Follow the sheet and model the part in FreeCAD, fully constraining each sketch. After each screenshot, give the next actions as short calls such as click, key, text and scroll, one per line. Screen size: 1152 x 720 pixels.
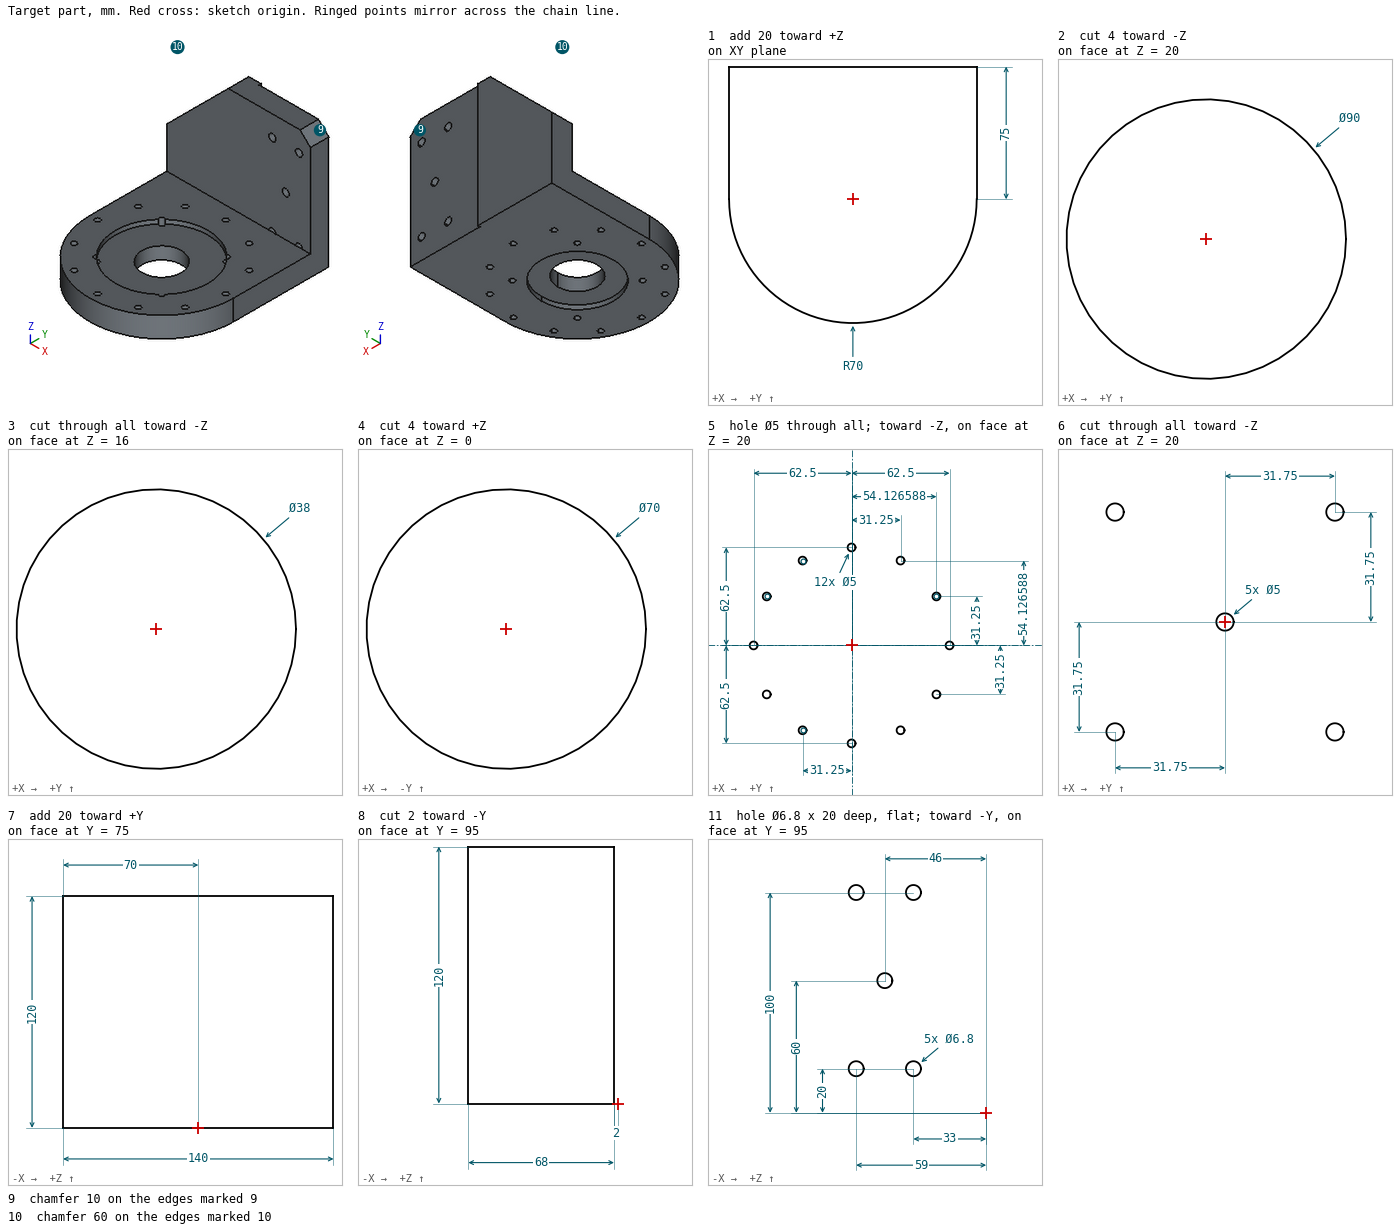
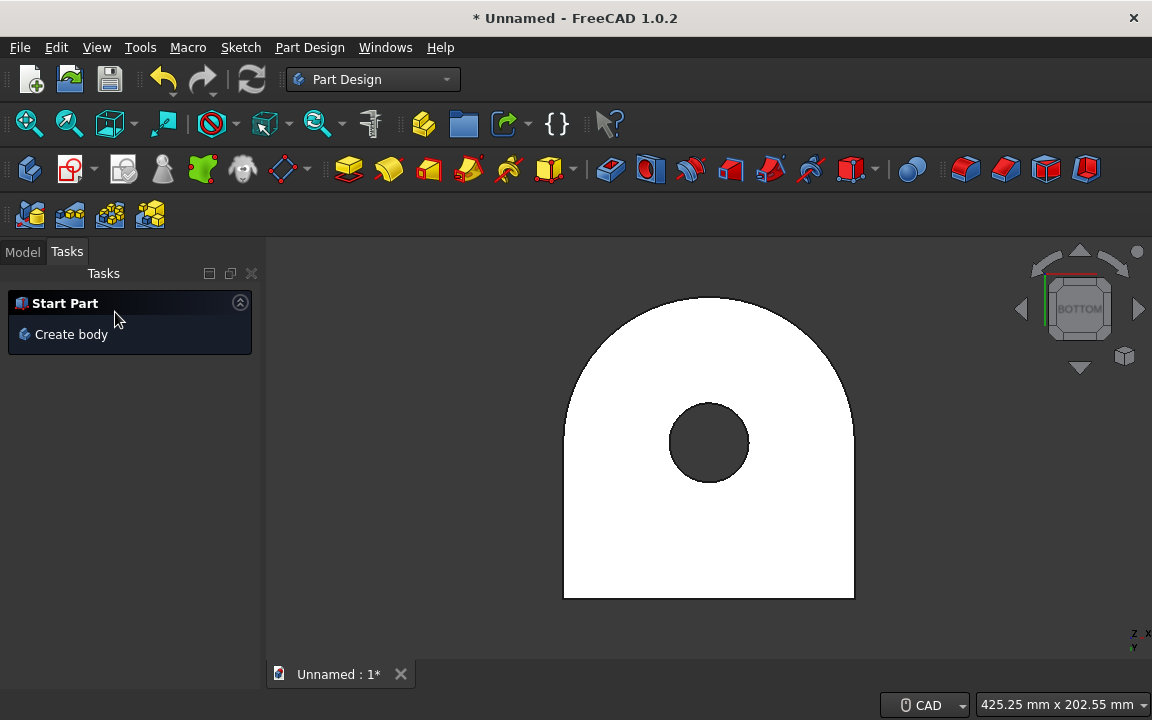
click(792, 533)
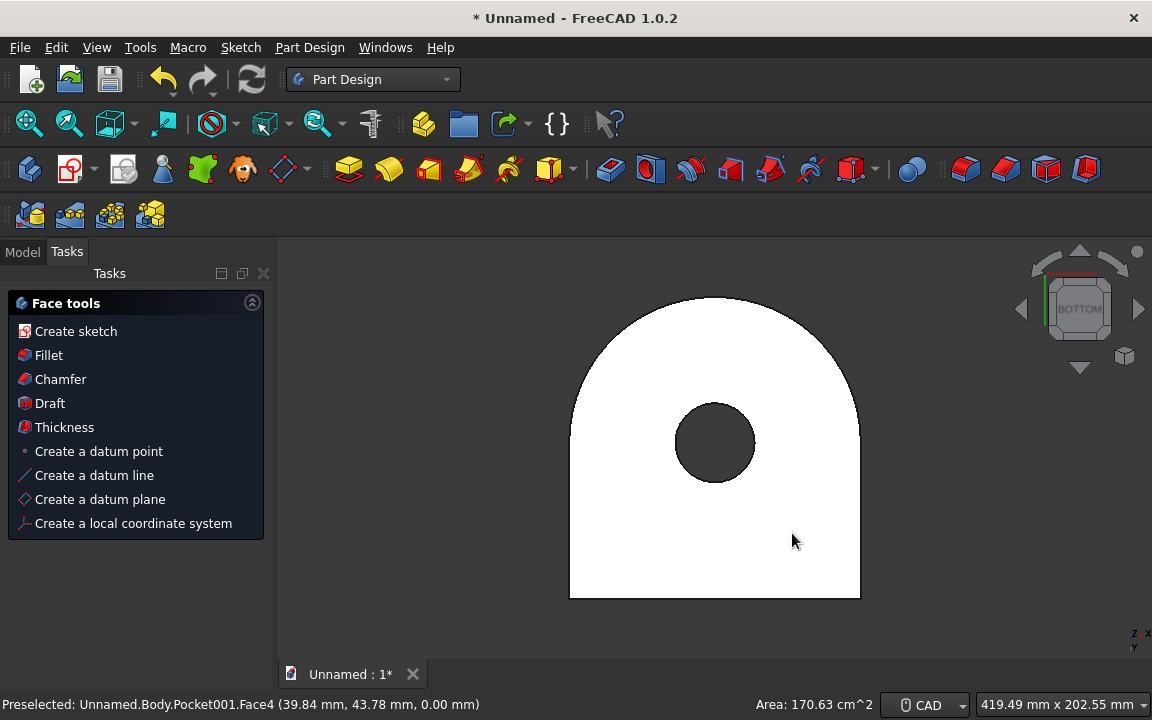
click(70, 170)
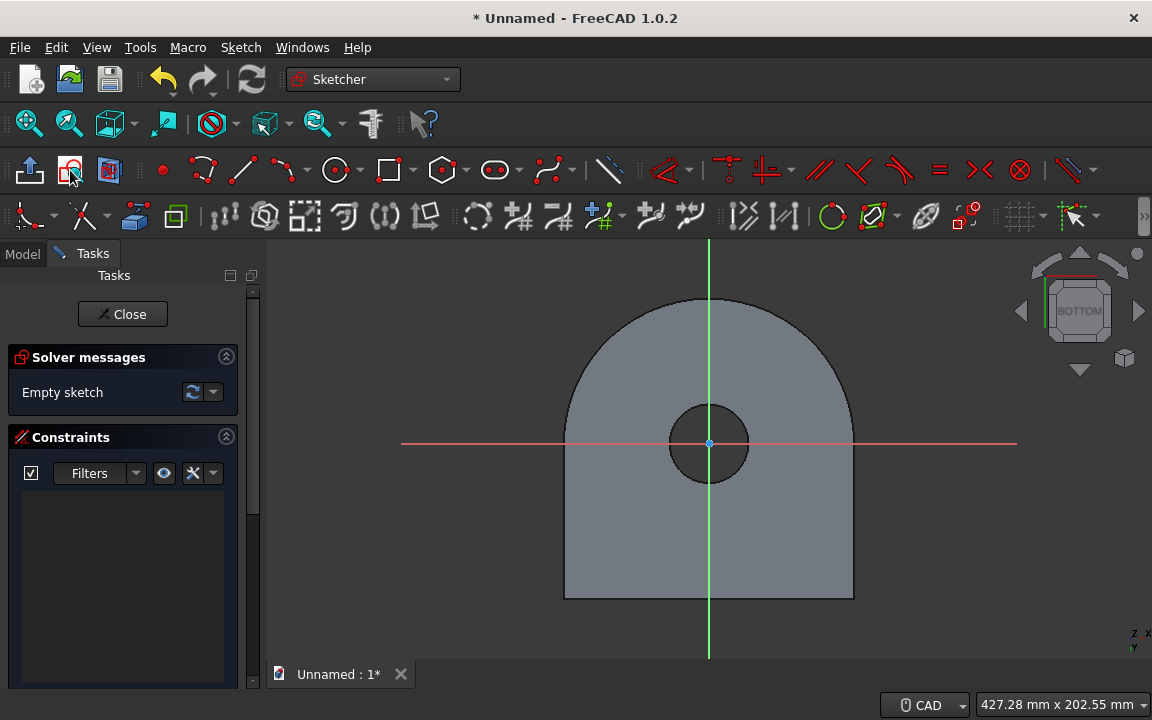
scroll(792, 438, up, 3)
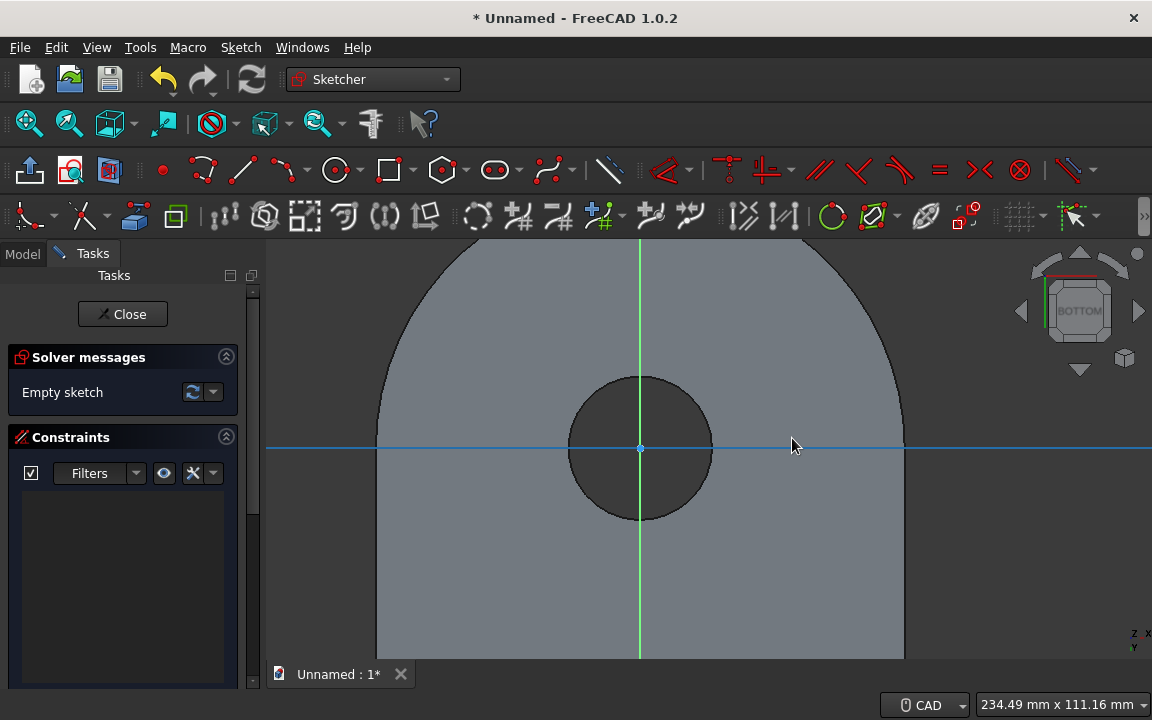
key(g)
key(c)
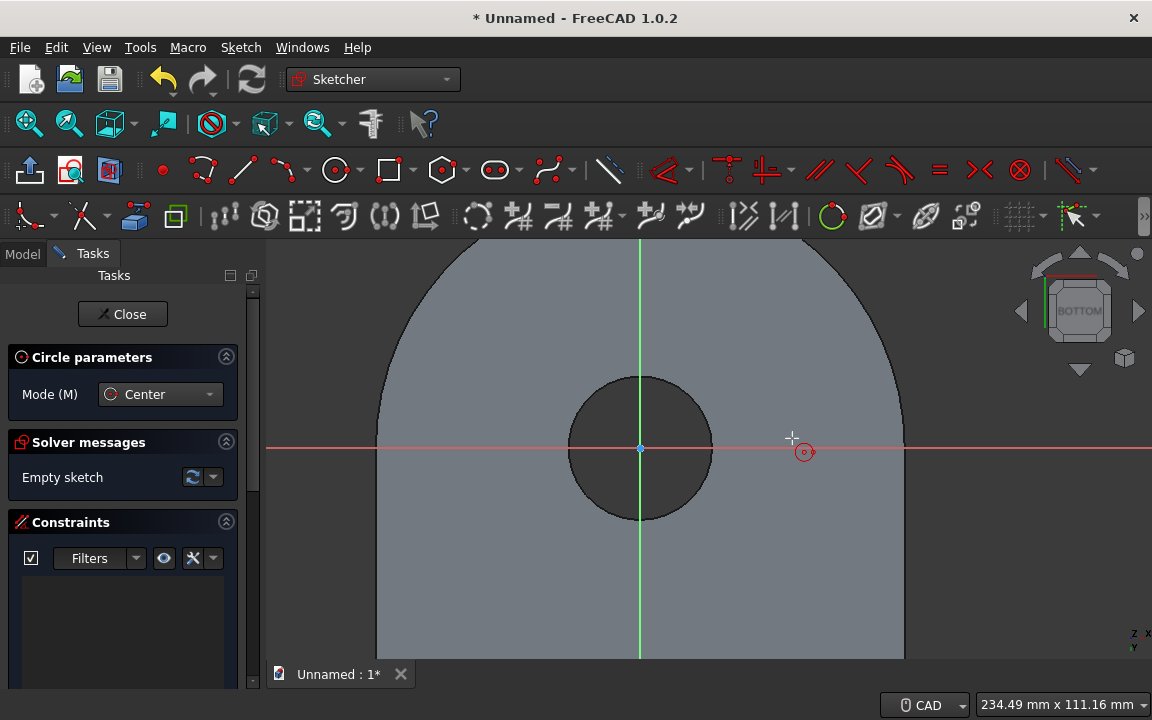
click(640, 448)
move(734, 355)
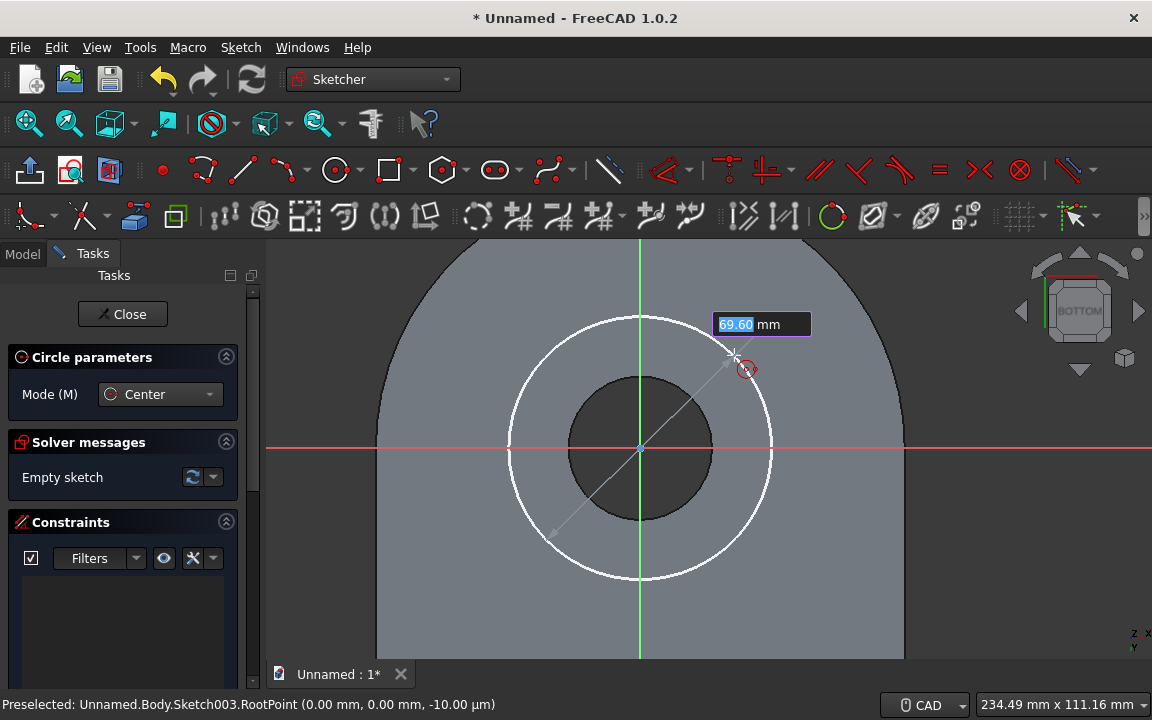
text(70)
key(Return)
key(Escape)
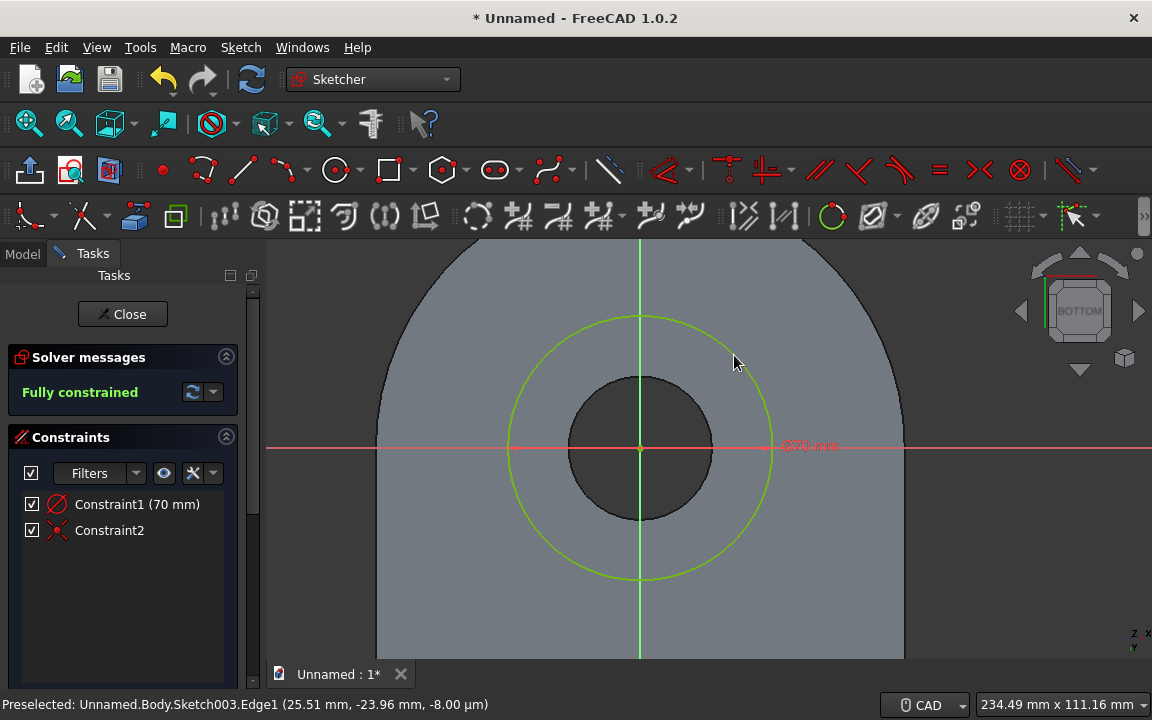
click(123, 314)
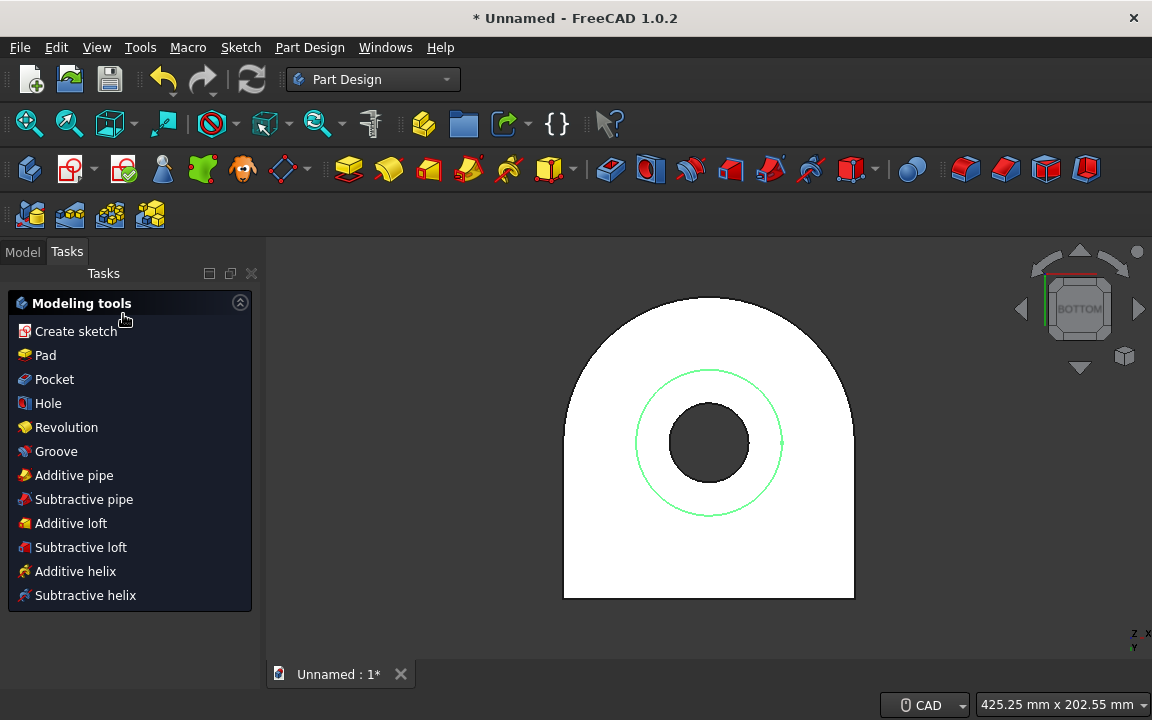
click(612, 170)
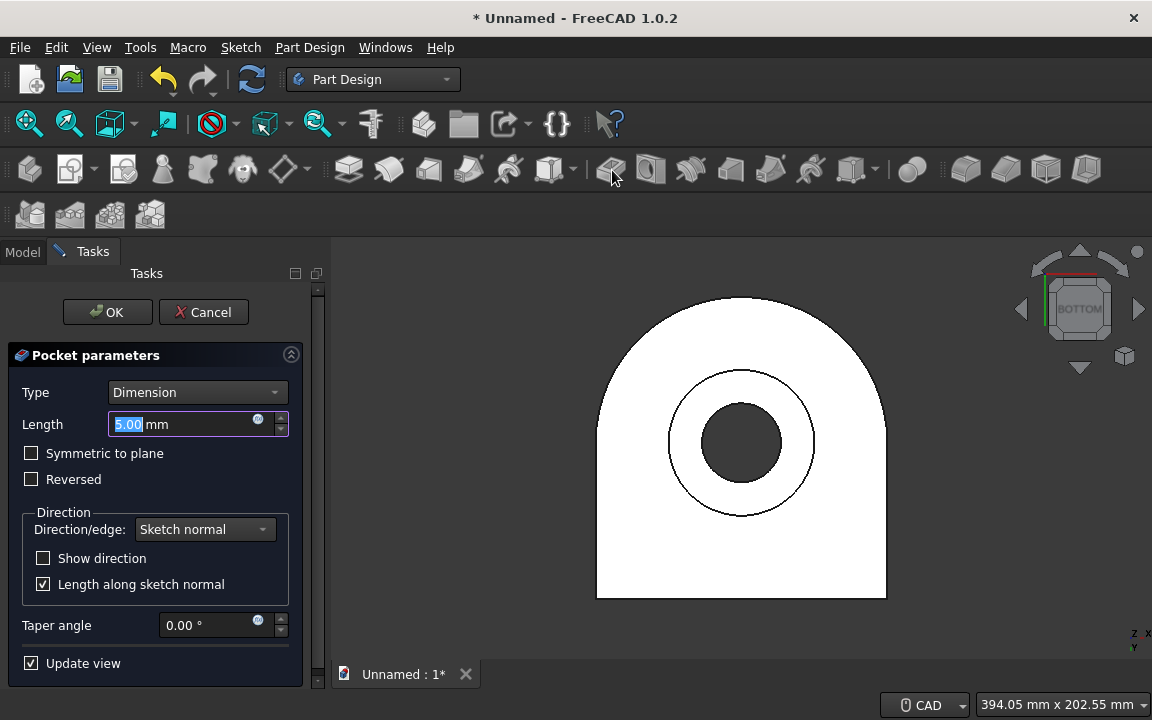
text(4)
key(Tab)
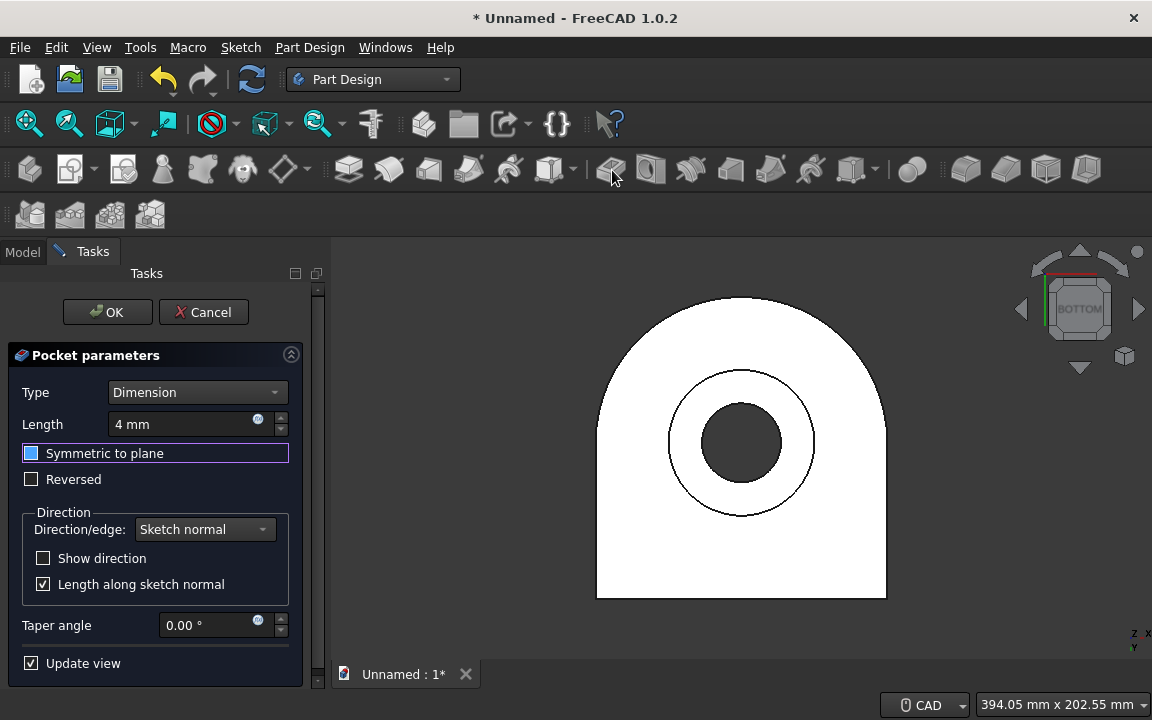
click(108, 312)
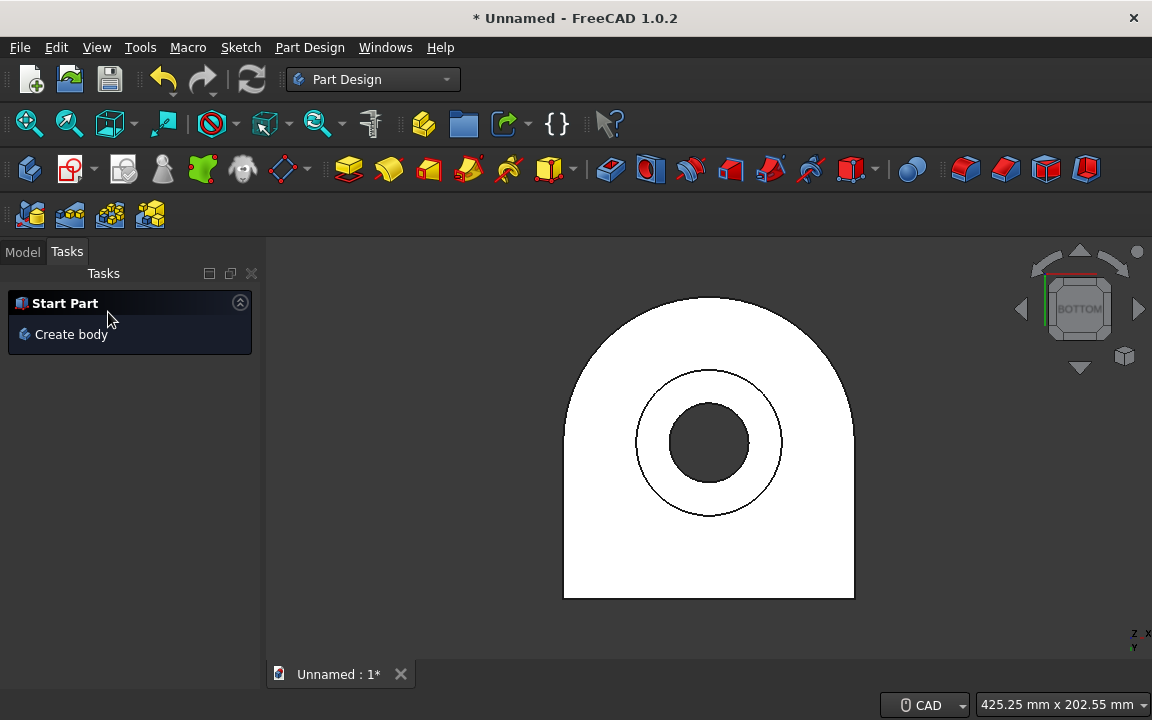
key(0)